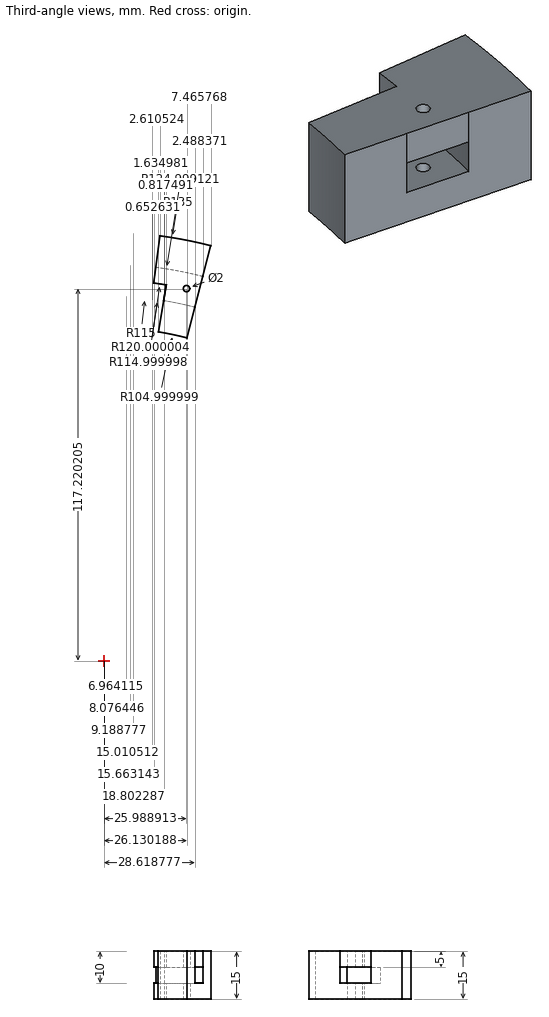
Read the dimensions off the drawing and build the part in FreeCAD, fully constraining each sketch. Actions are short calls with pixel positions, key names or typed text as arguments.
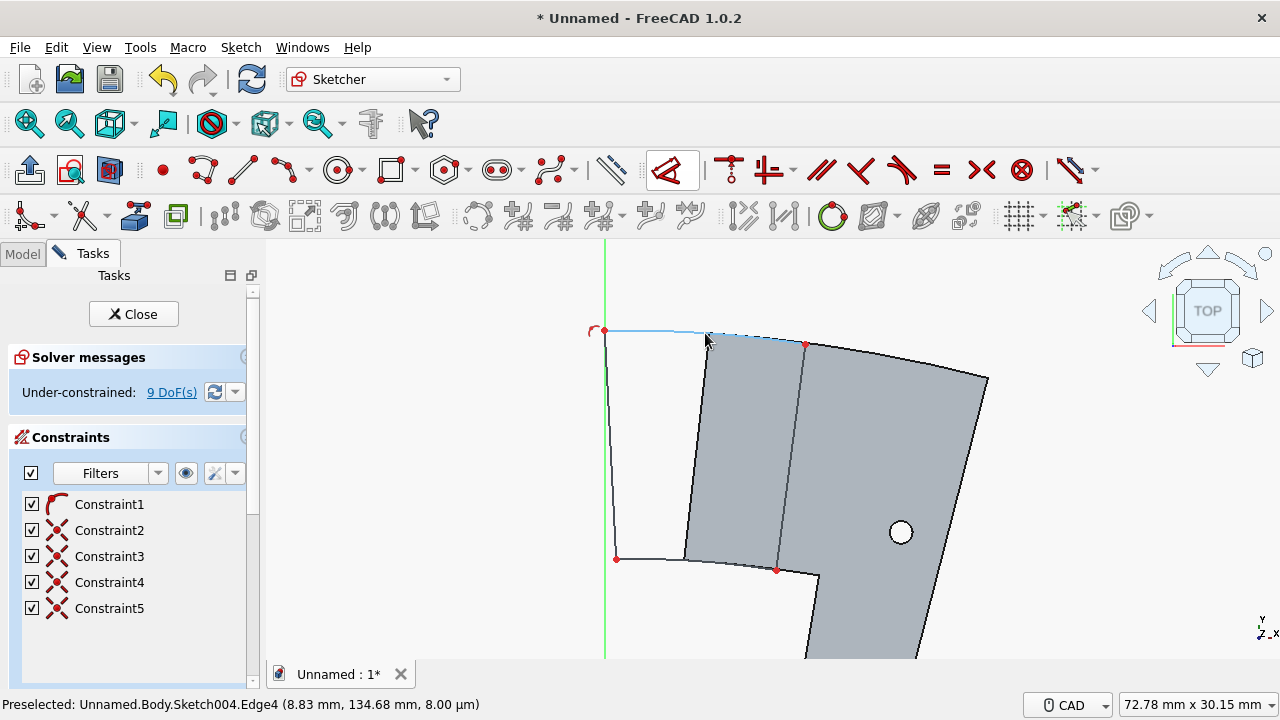
scroll(608, 399, up, 7)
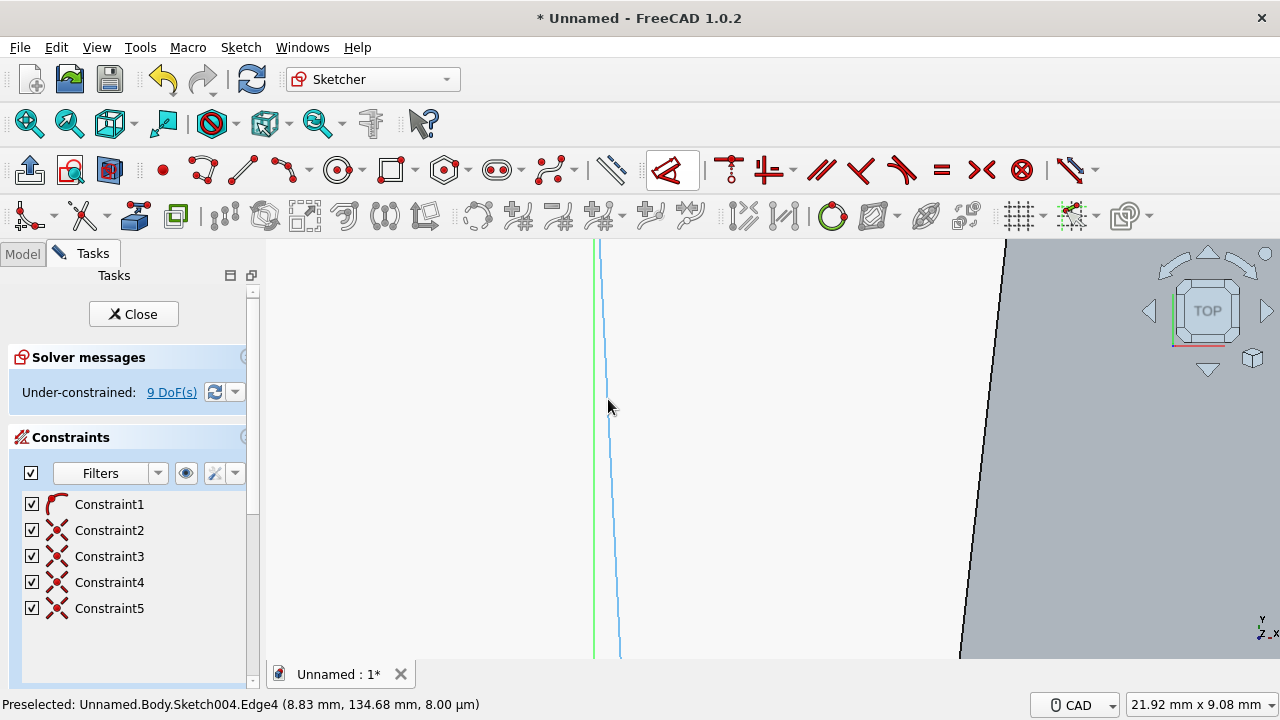
click(608, 399)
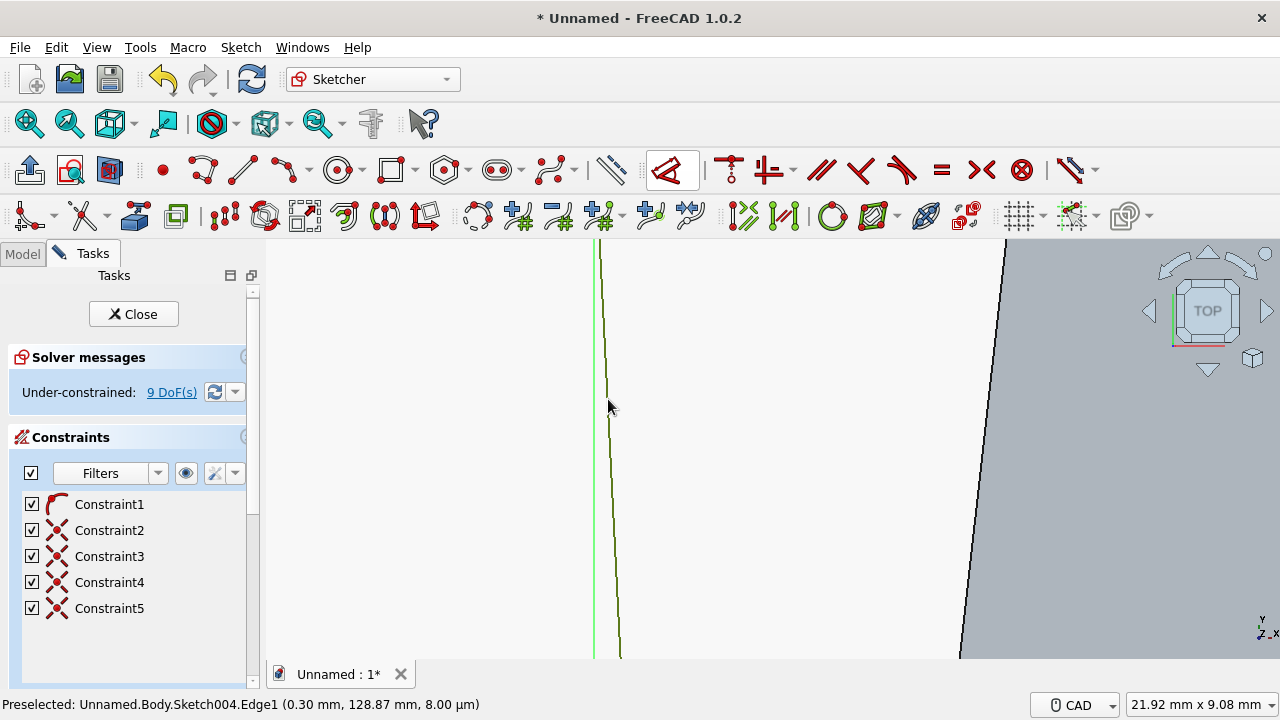
key(v)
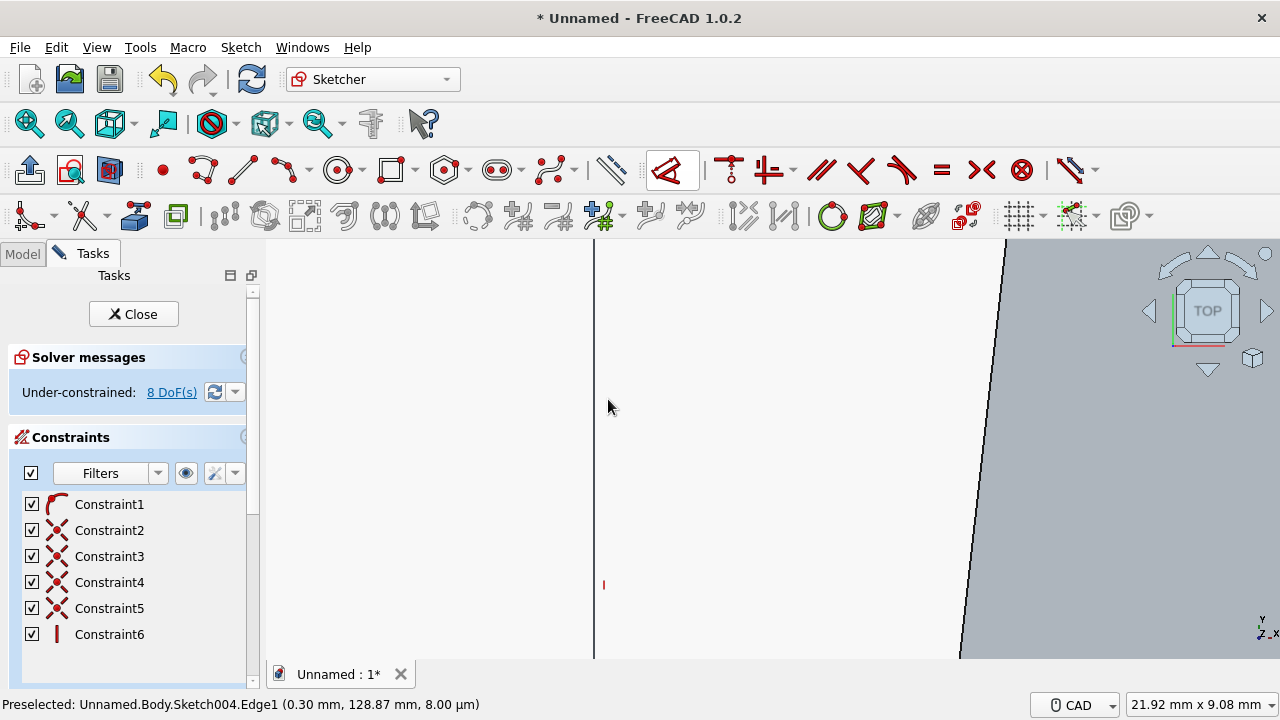
scroll(607, 399, down, 7)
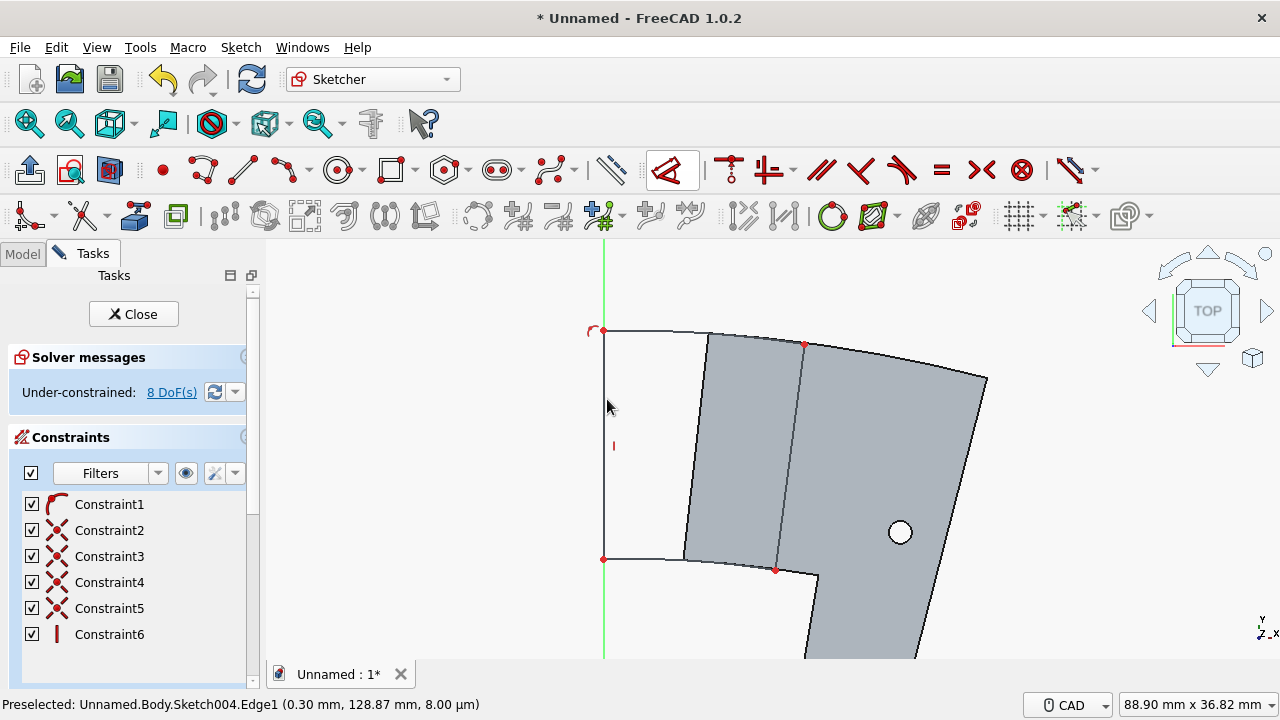
click(724, 563)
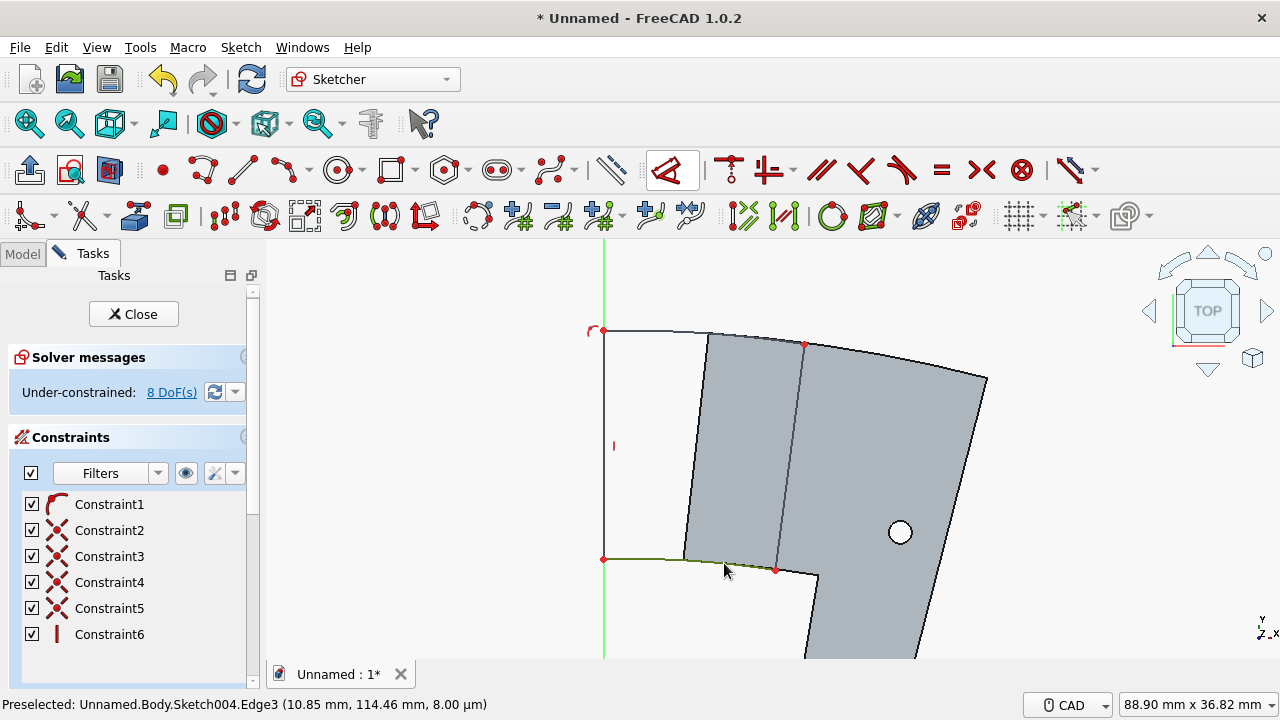
click(745, 337)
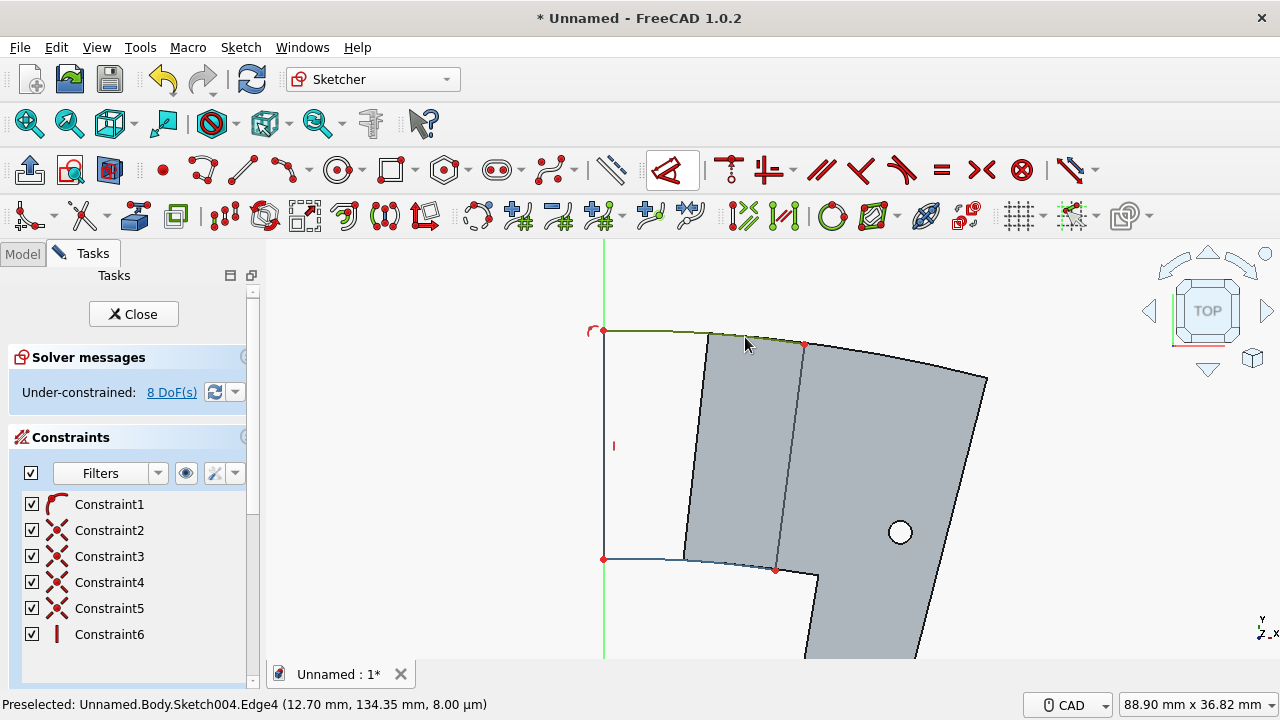
click(730, 170)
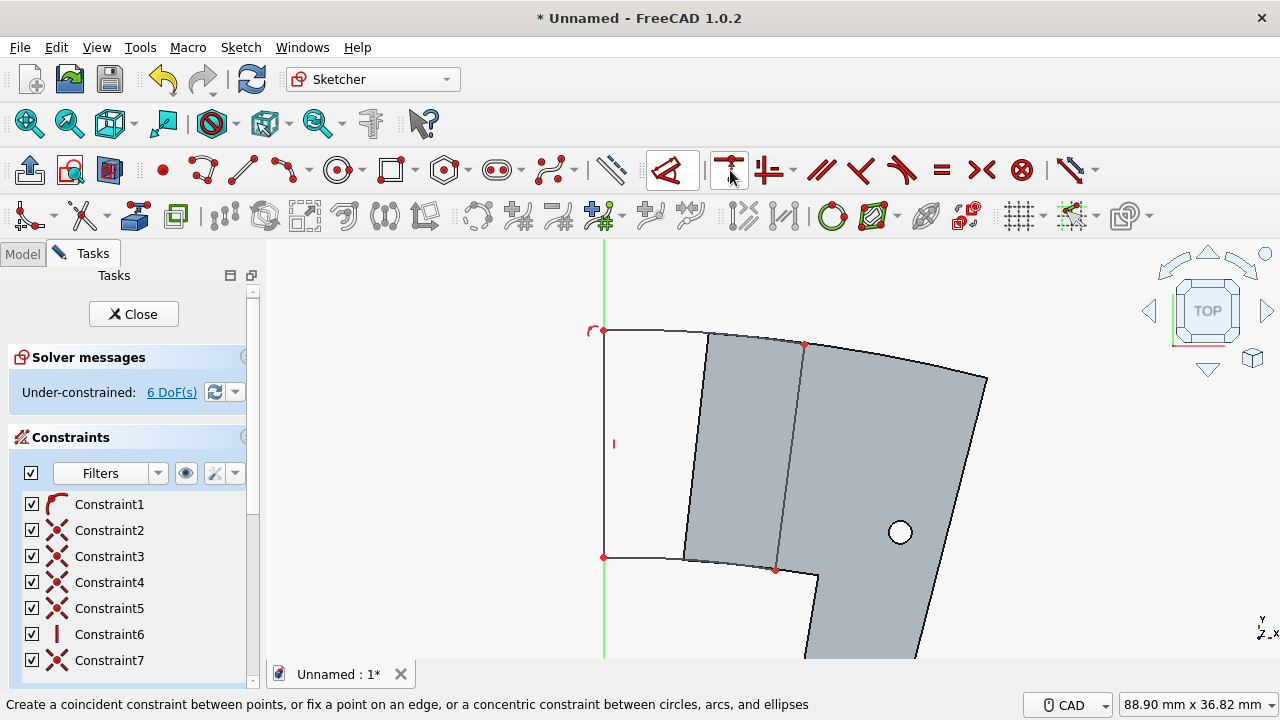
scroll(705, 311, down, 8)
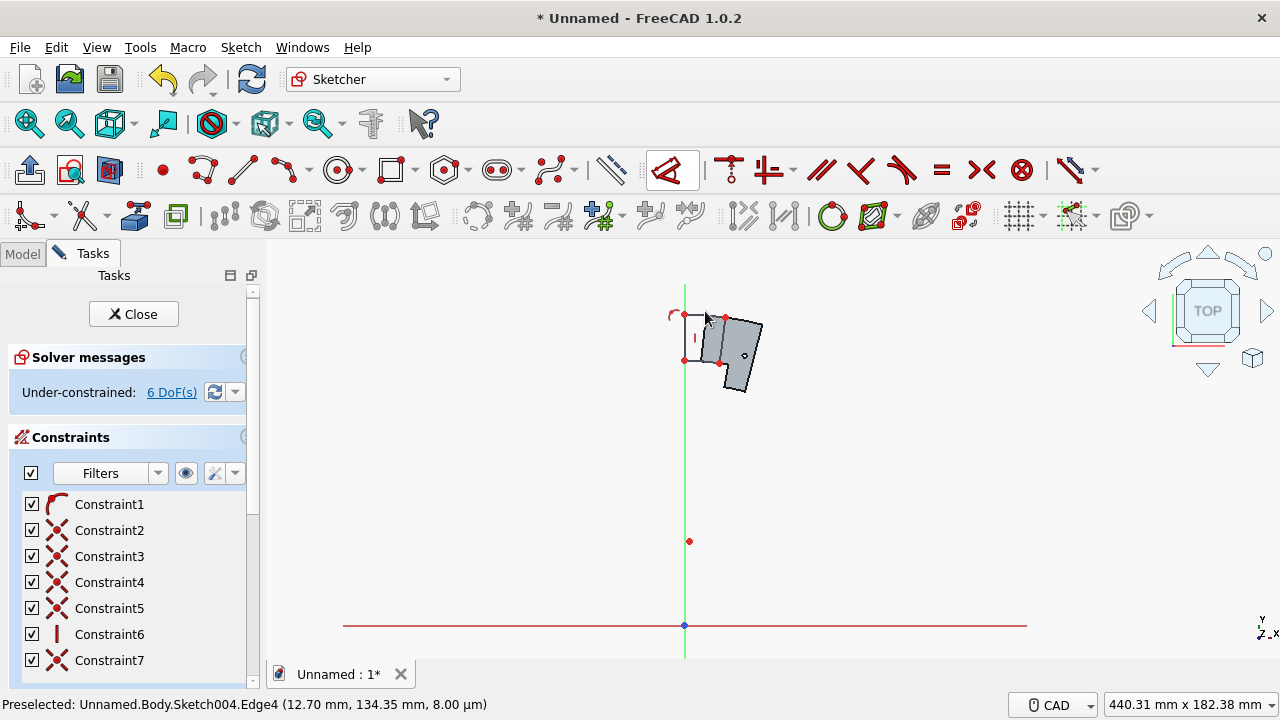
drag(675, 531, 699, 636)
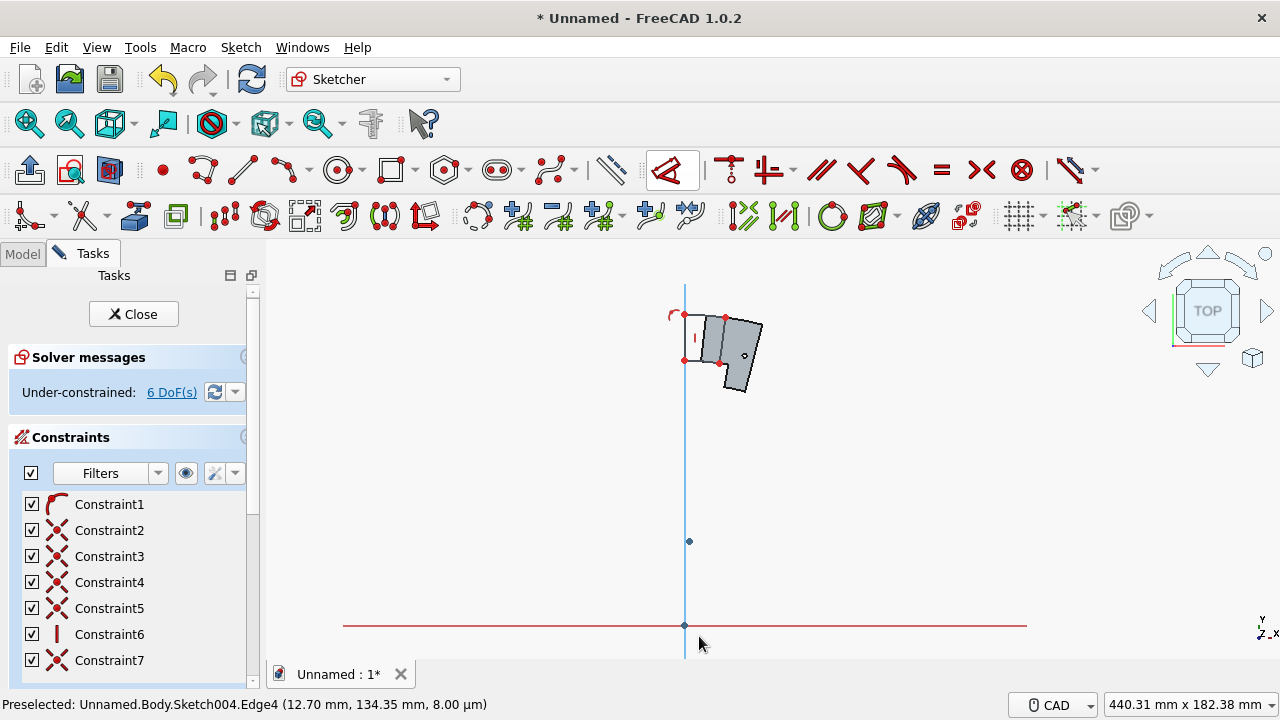
click(730, 170)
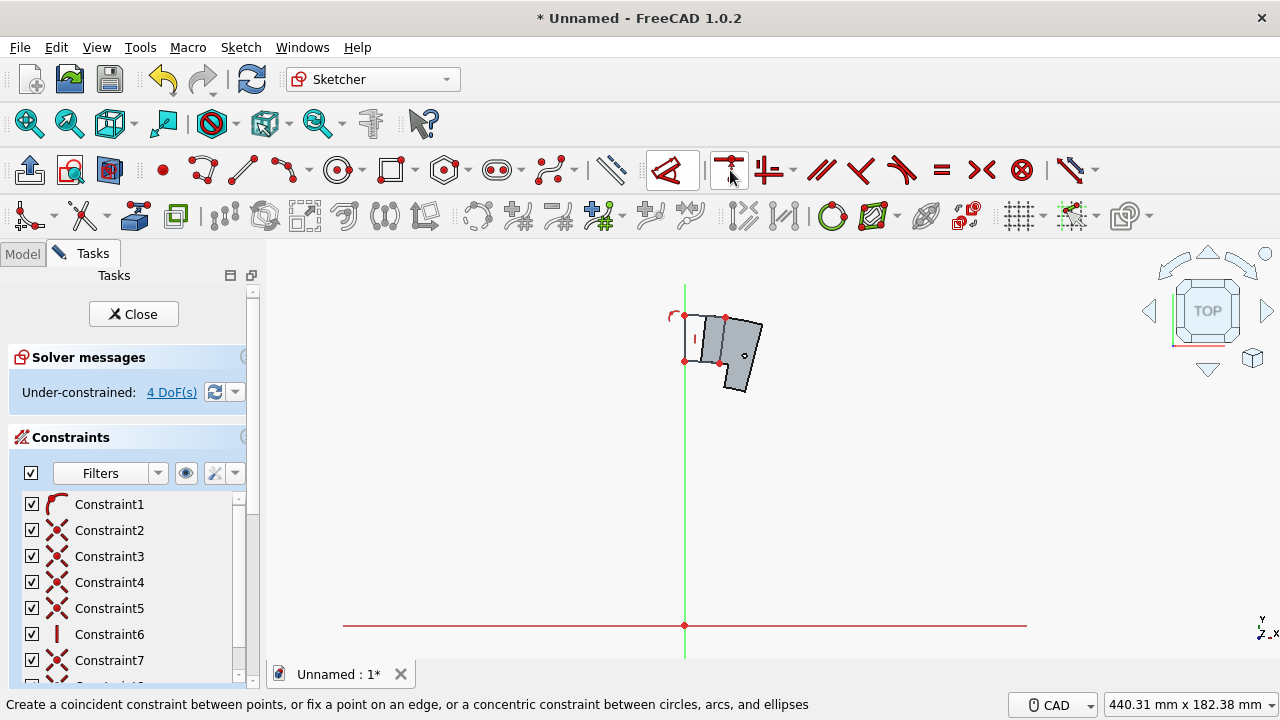
scroll(709, 362, up, 2)